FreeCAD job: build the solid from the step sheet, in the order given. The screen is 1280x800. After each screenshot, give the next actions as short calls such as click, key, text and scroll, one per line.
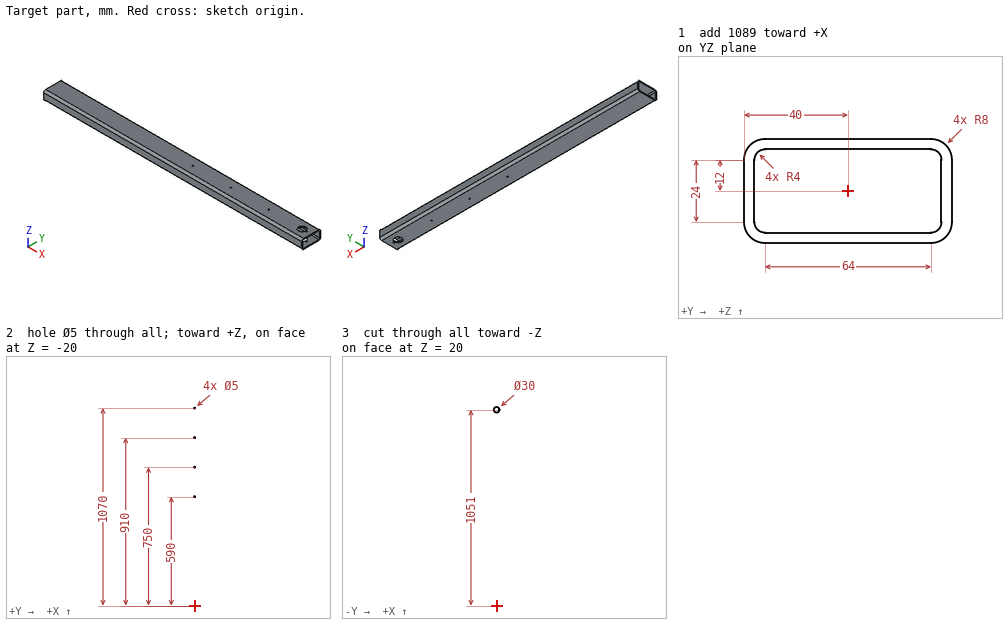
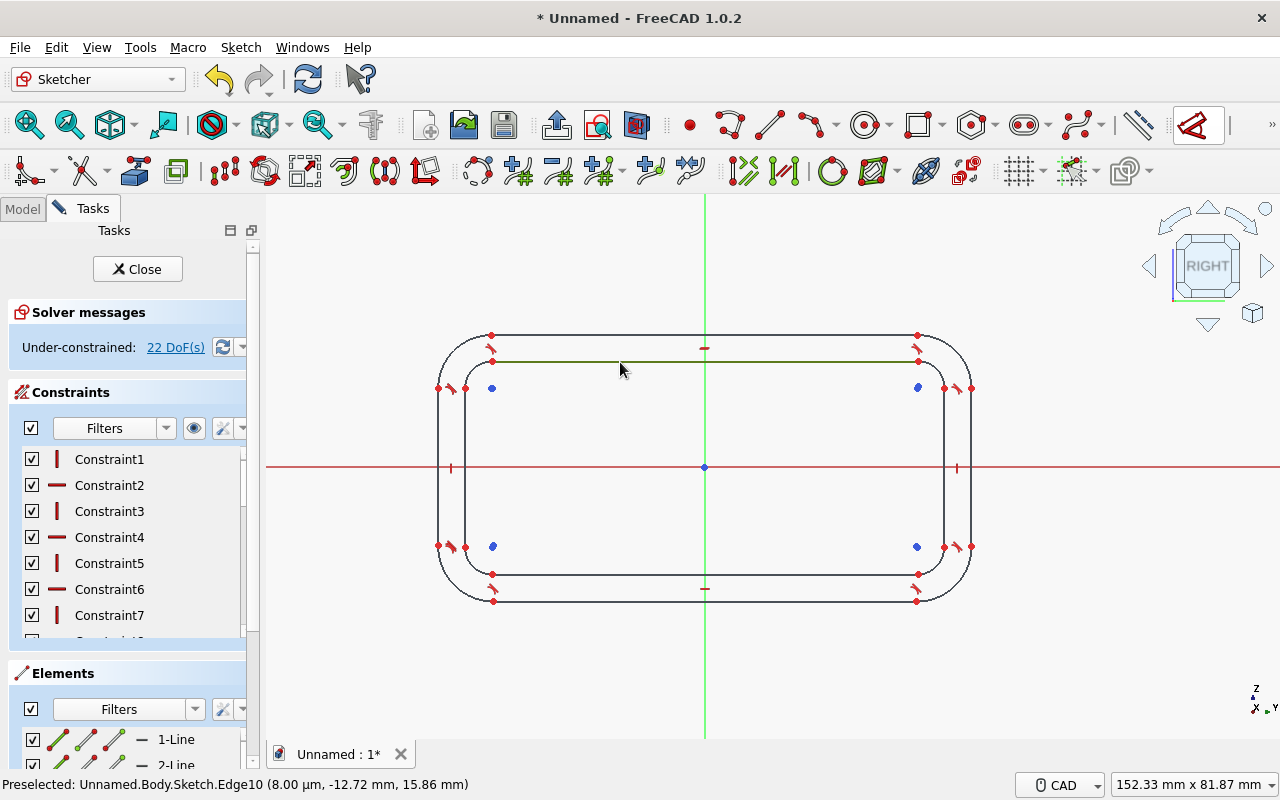
click(480, 364)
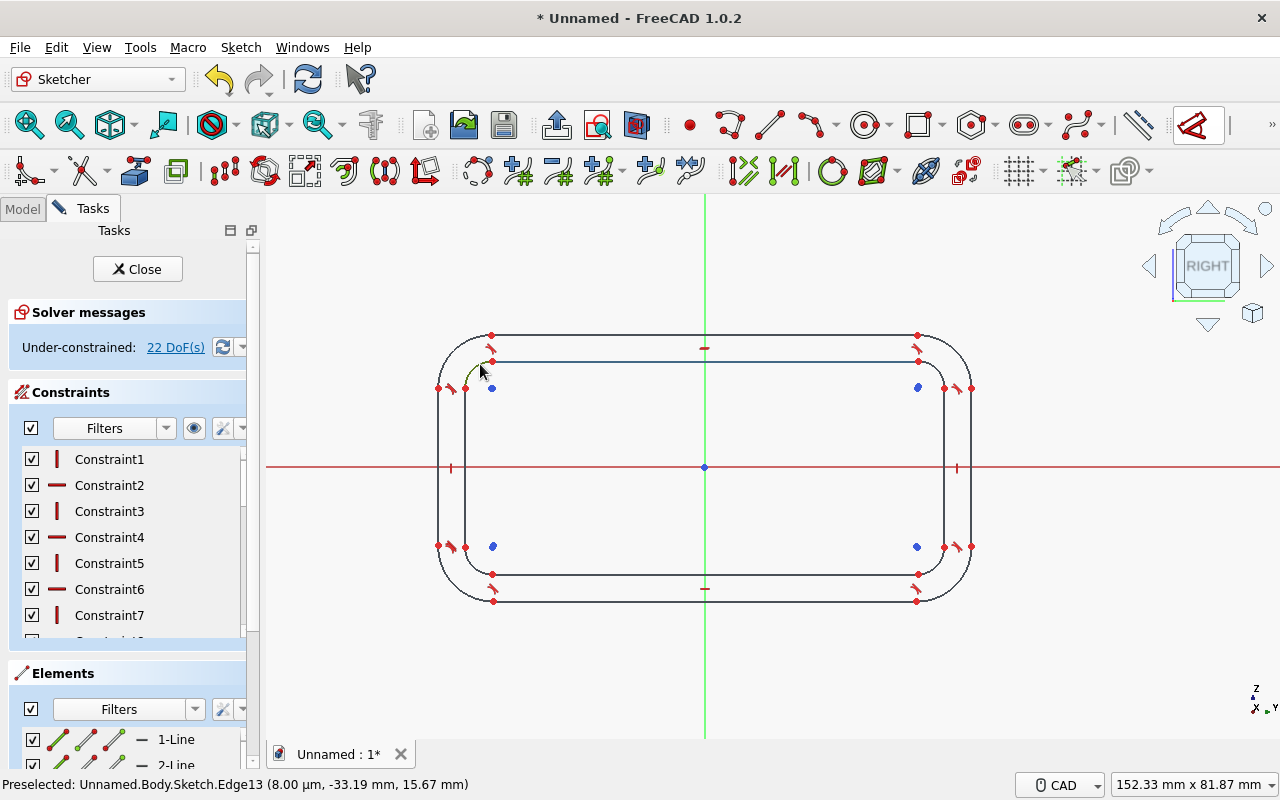
key(t)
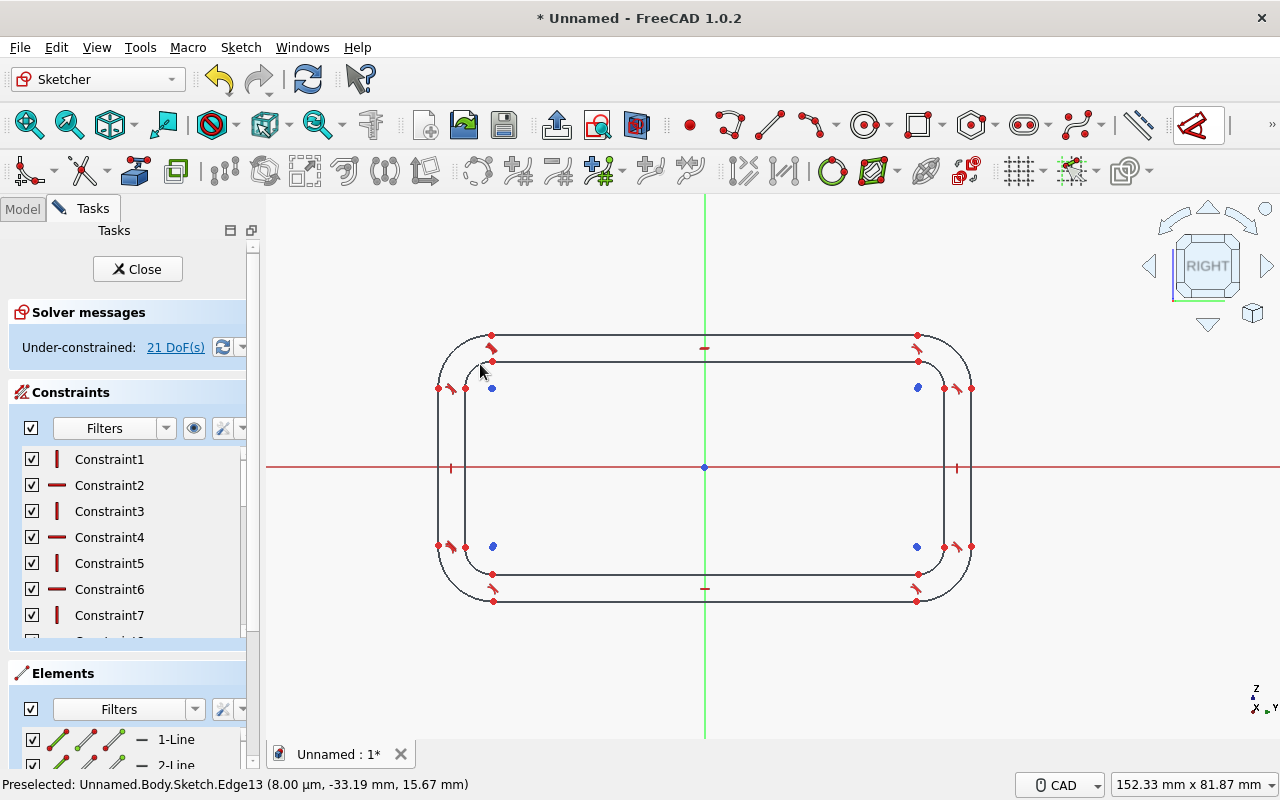
click(620, 362)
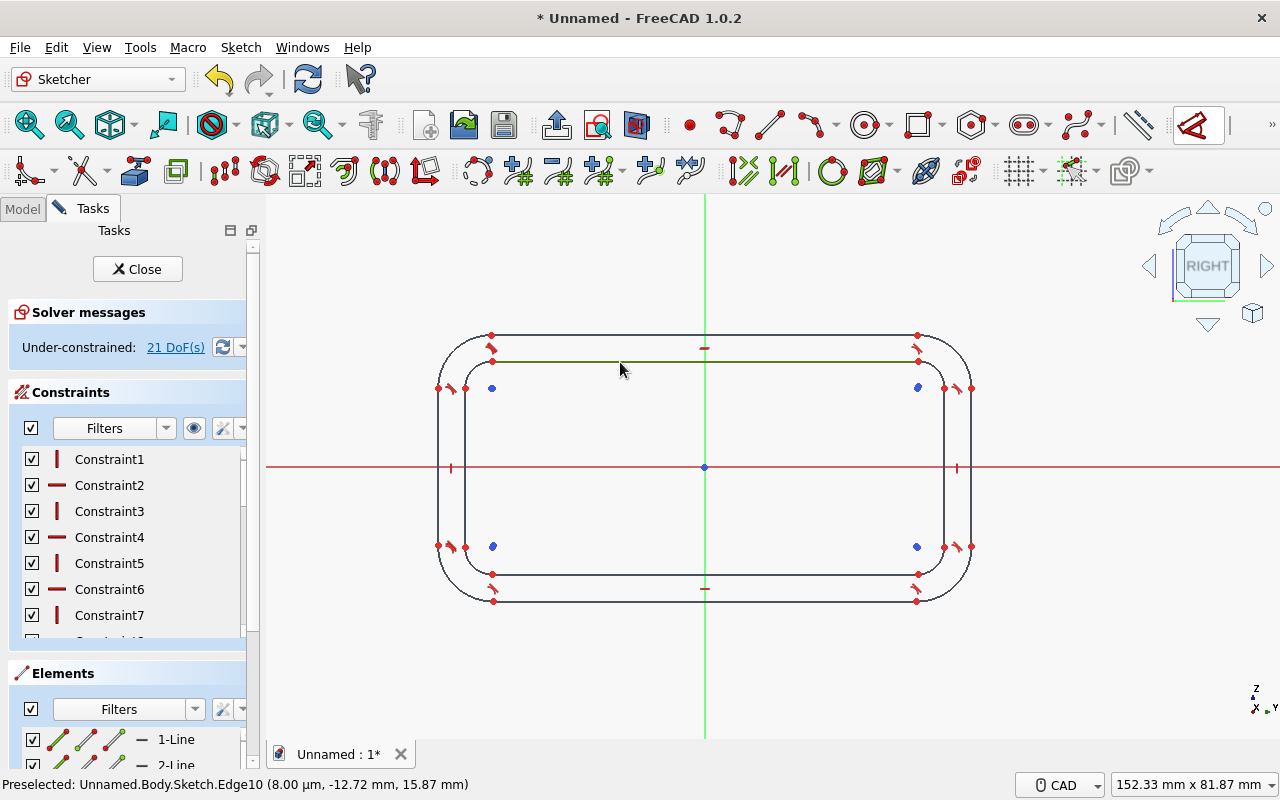
click(942, 376)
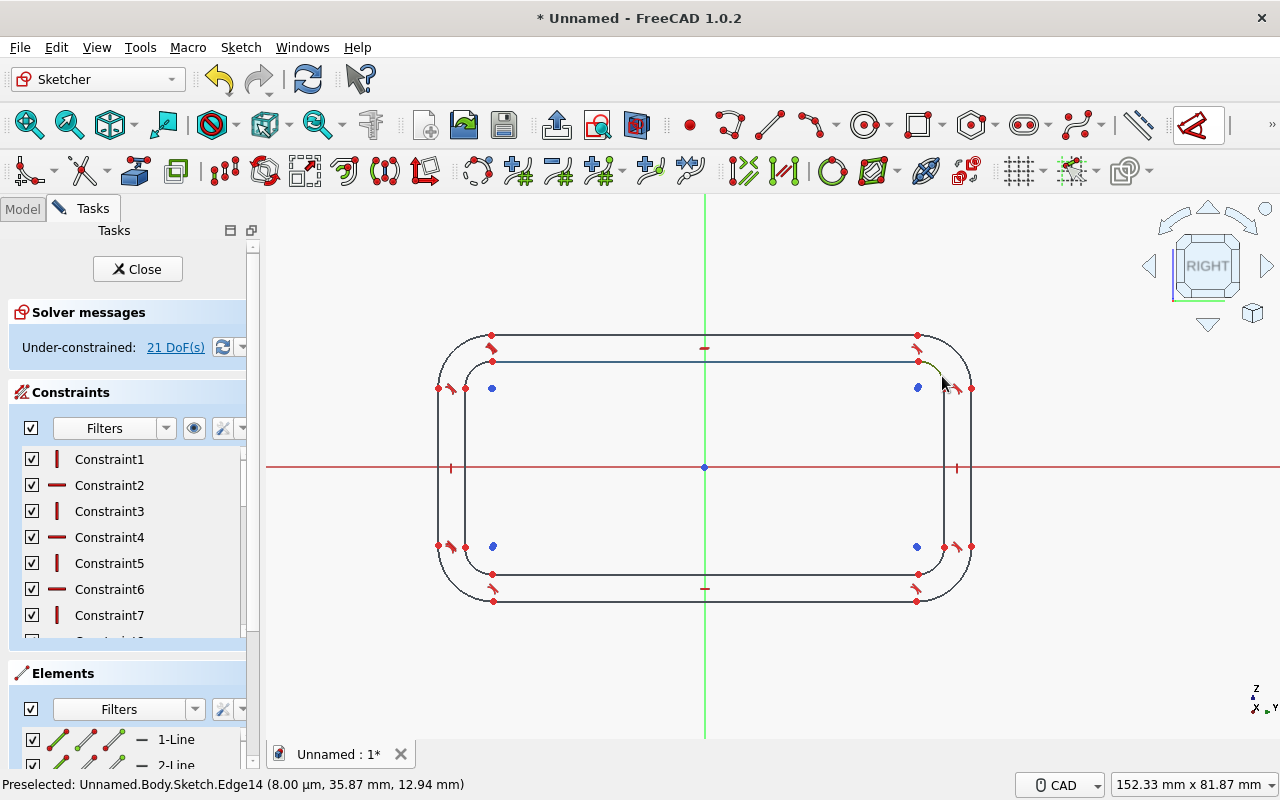
key(t)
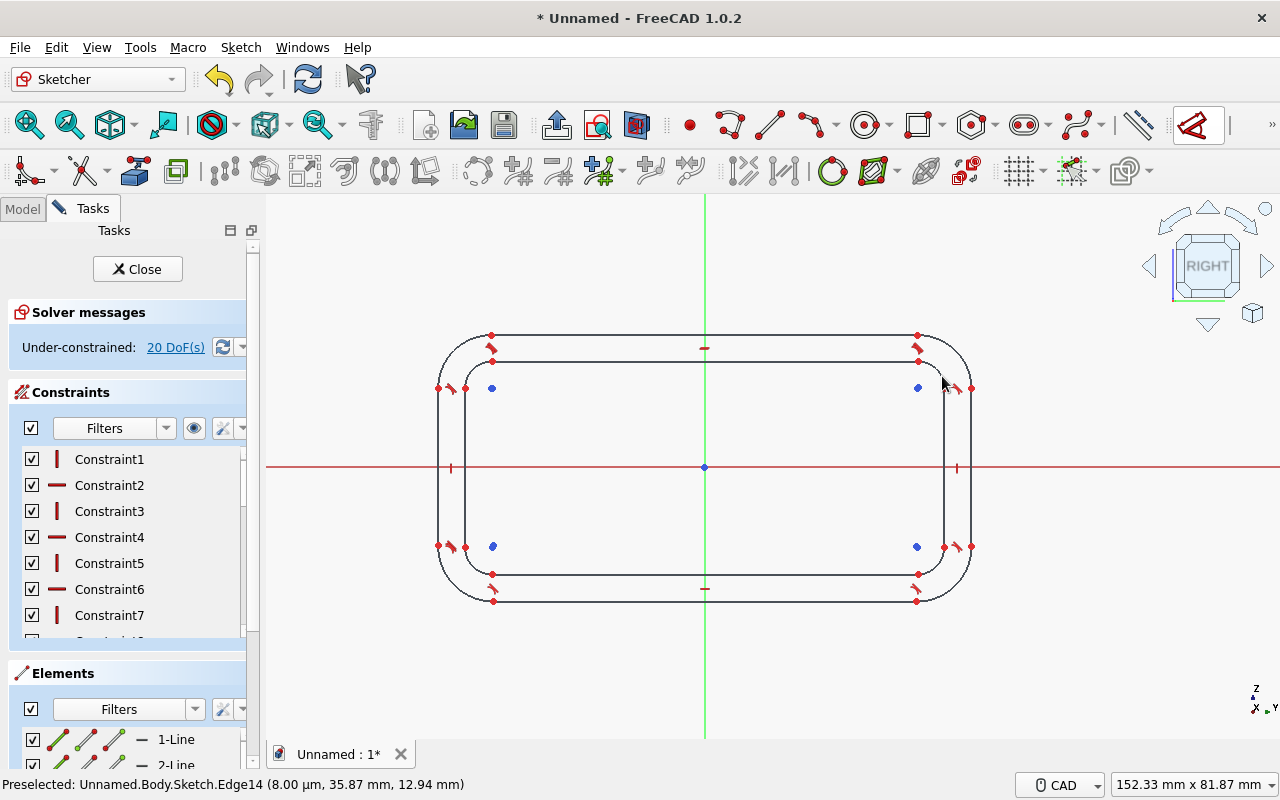
click(944, 436)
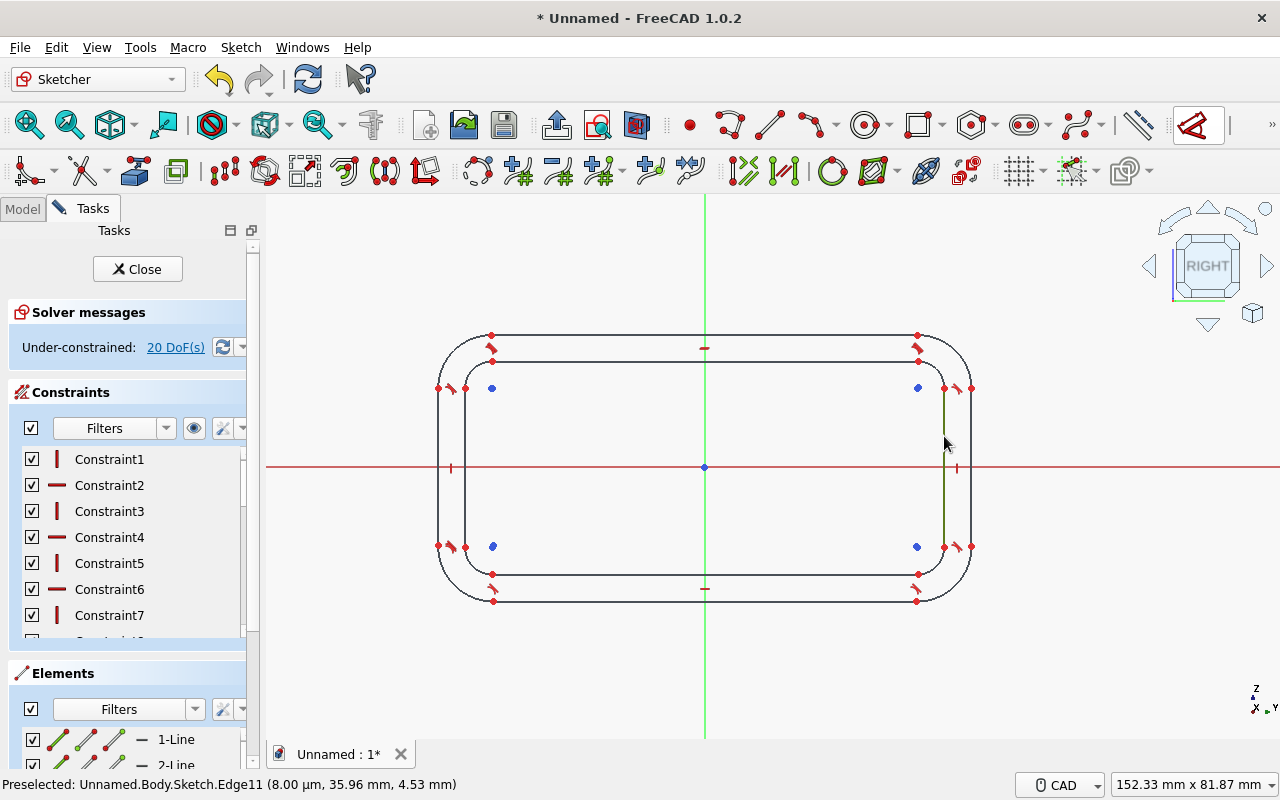
click(942, 376)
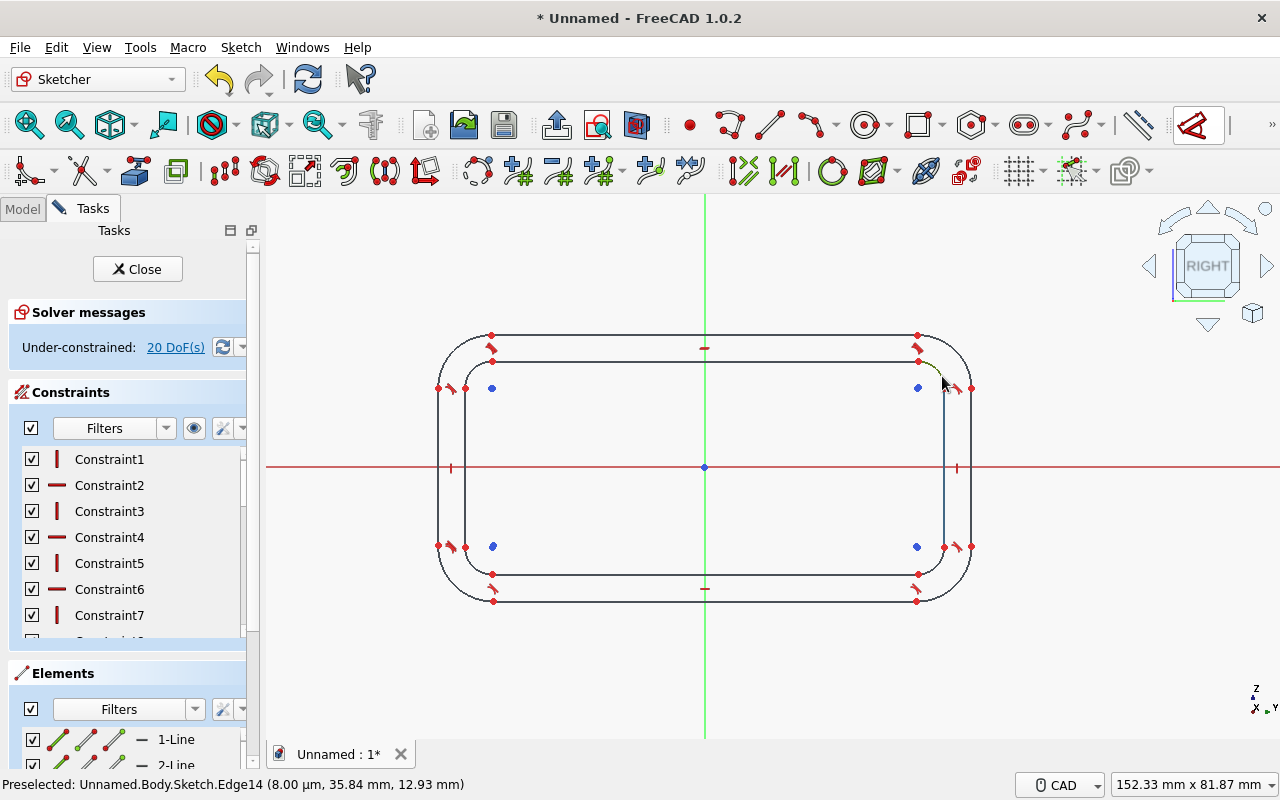
key(t)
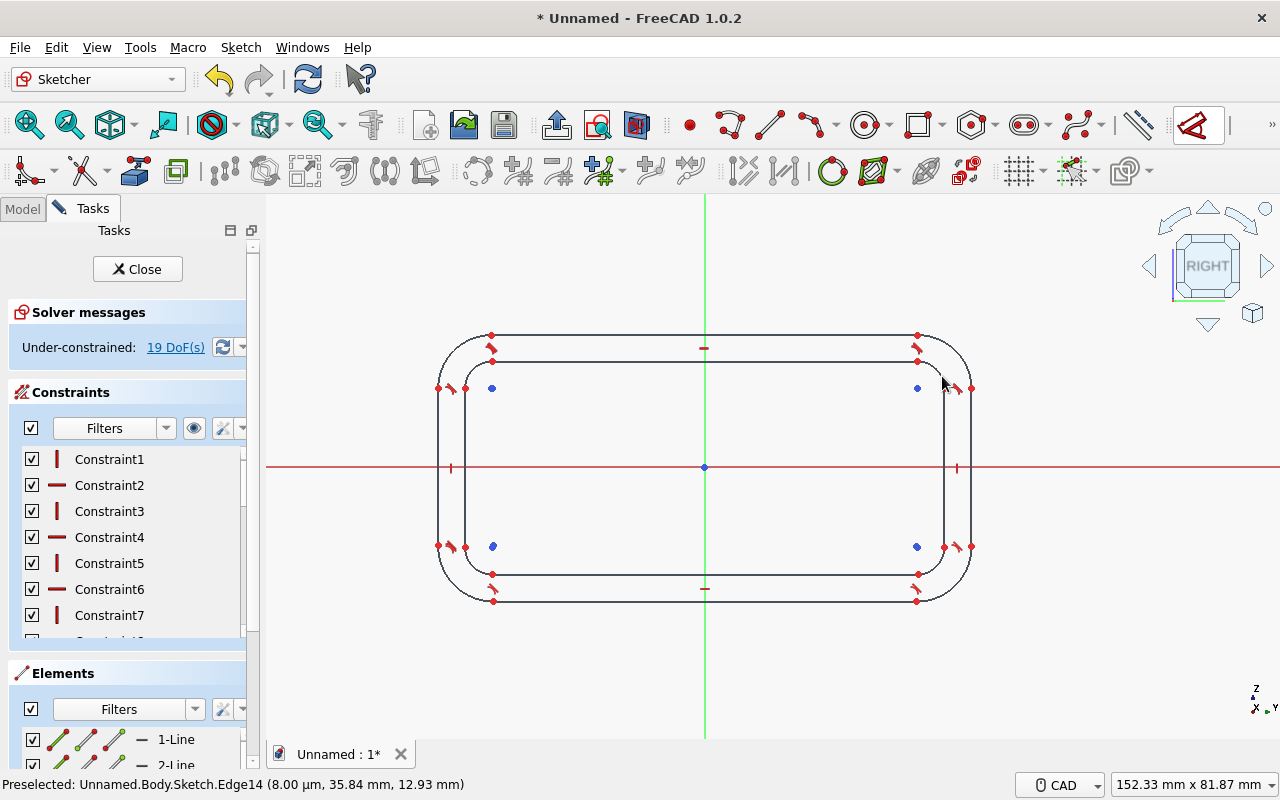
click(944, 436)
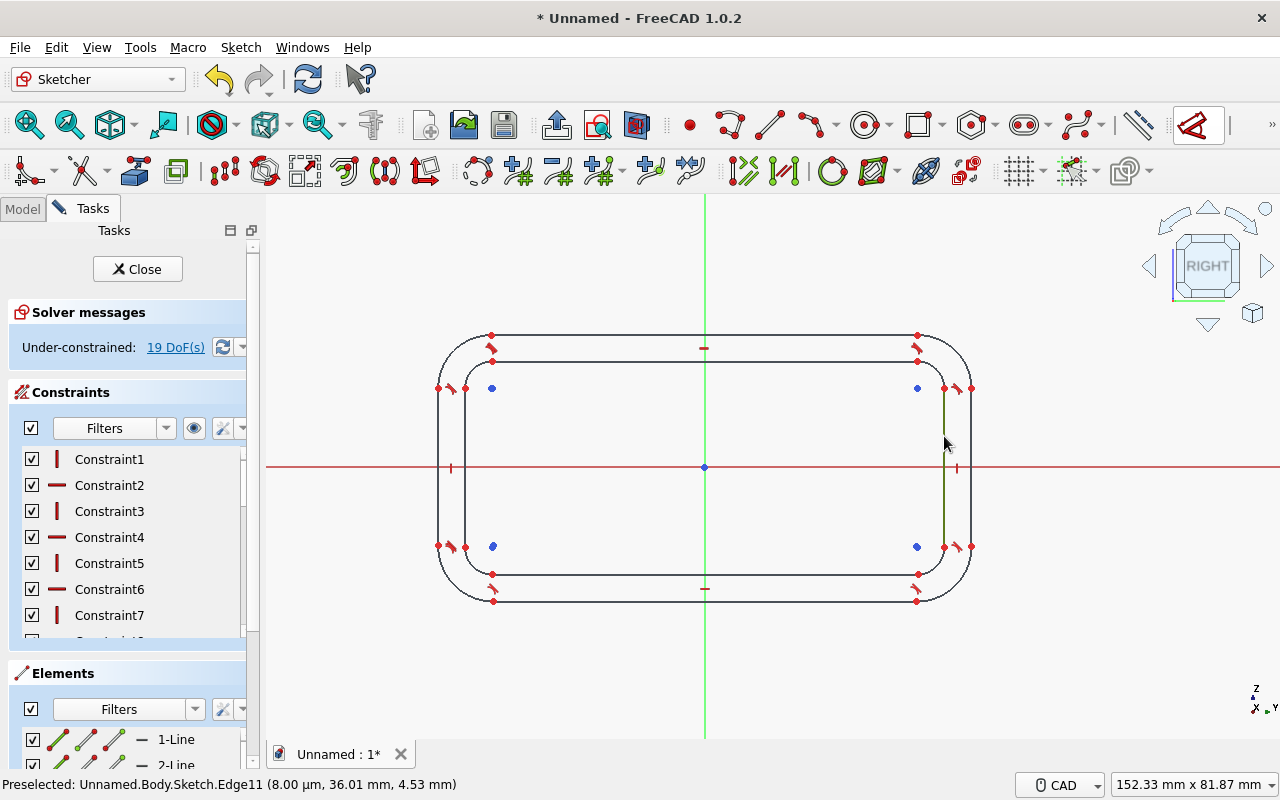
click(930, 571)